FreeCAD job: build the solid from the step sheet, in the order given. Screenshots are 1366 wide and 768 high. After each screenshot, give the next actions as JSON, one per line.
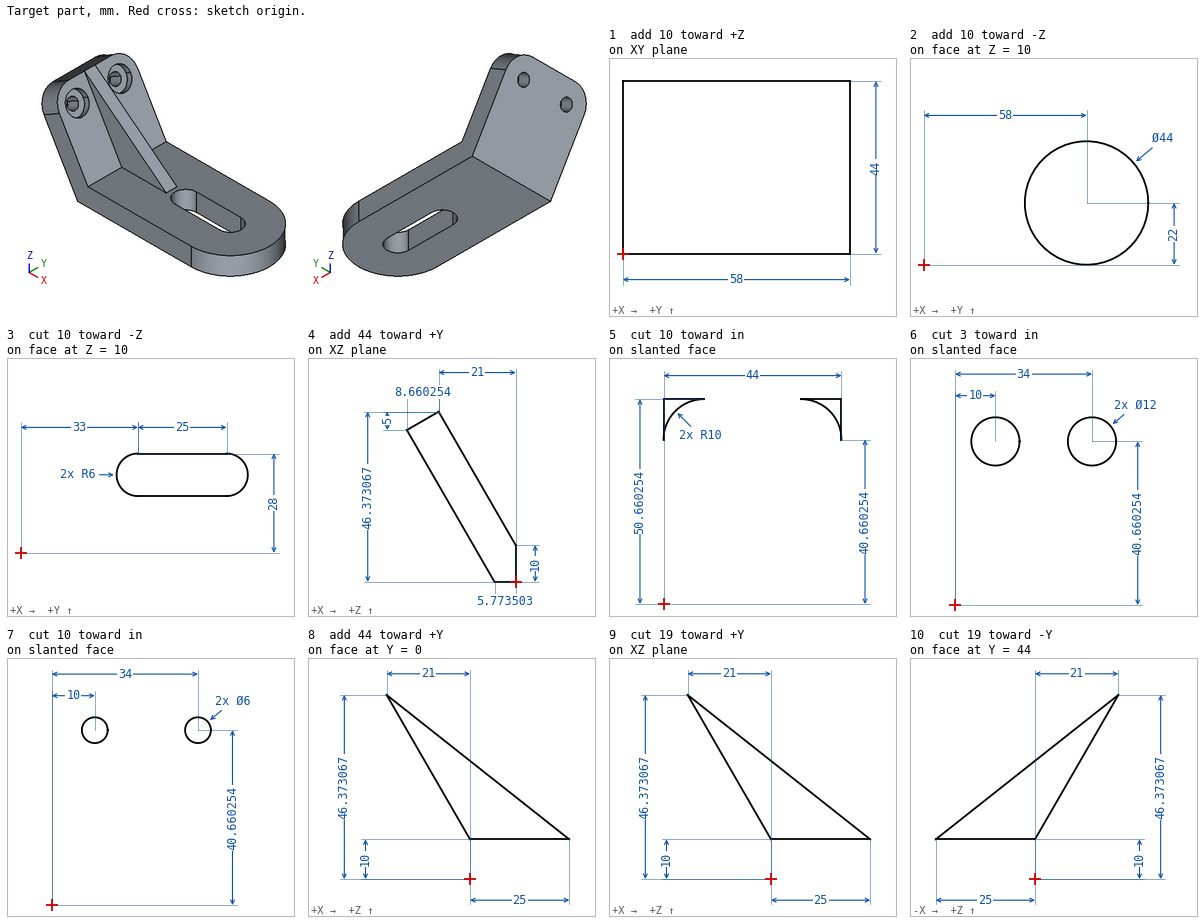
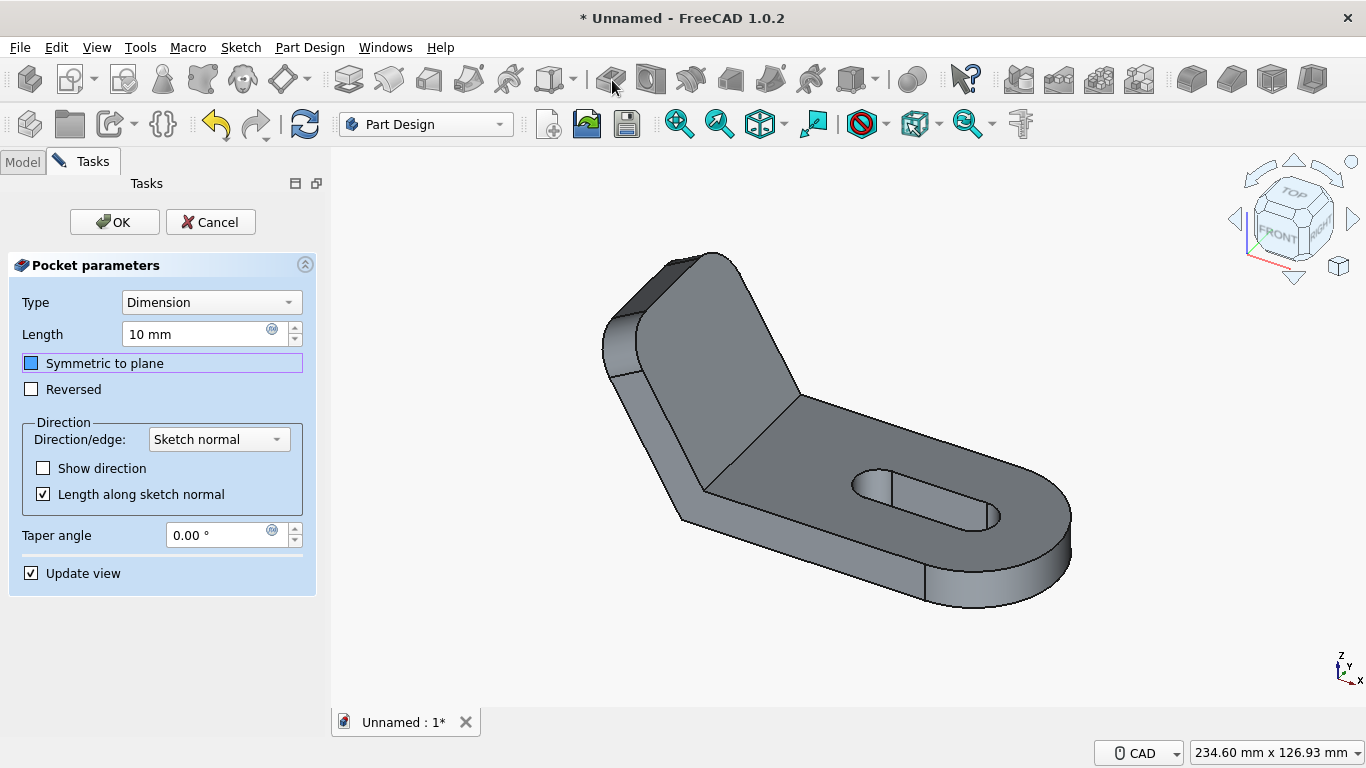
{"action": "left_click", "coordinate": [115, 222]}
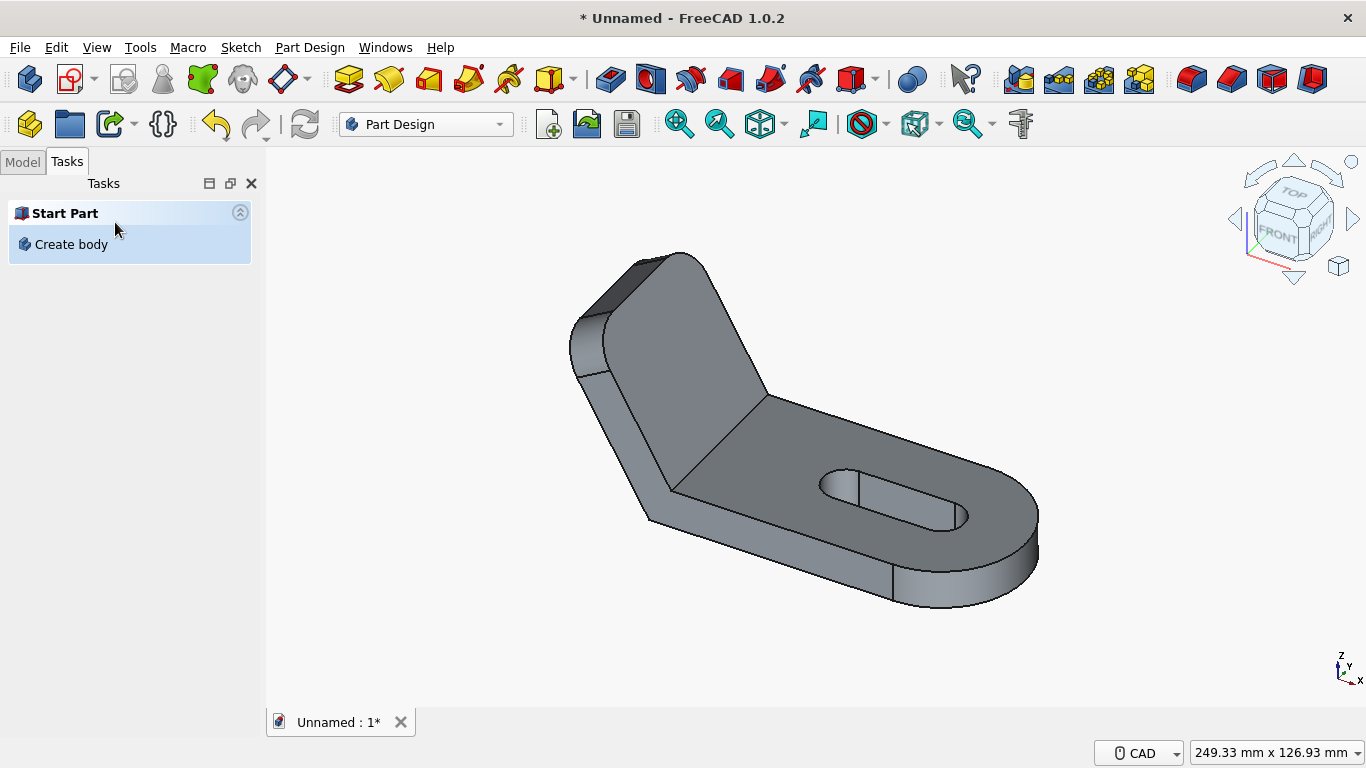
{"action": "left_click", "coordinate": [680, 363]}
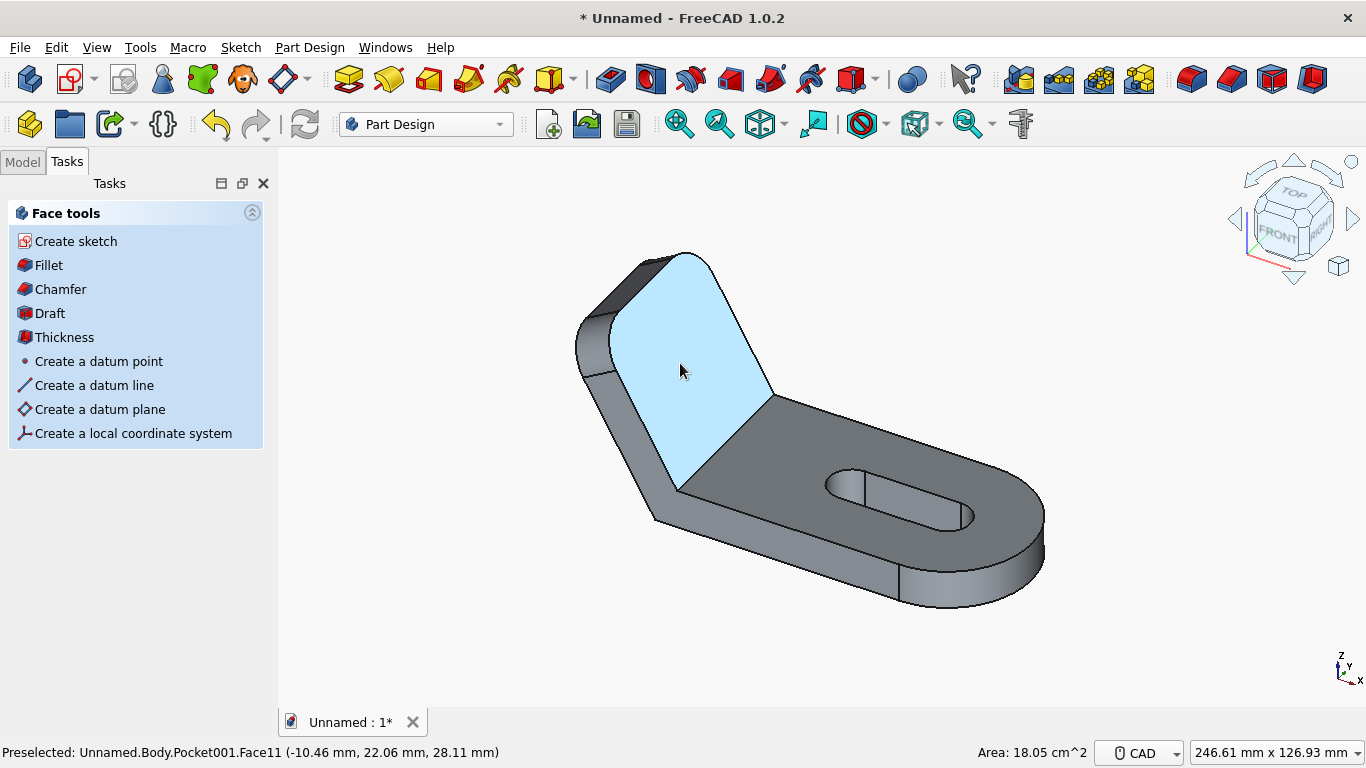
{"action": "left_click", "coordinate": [70, 80]}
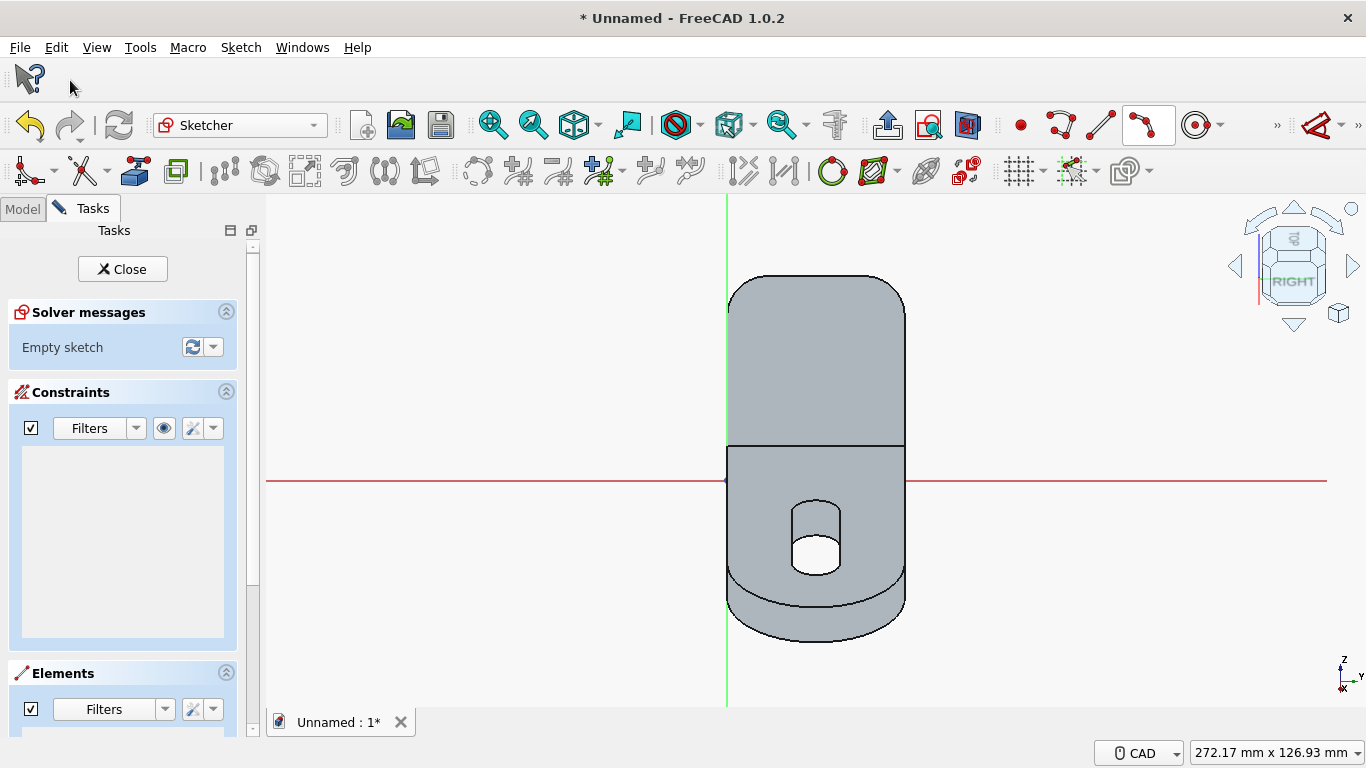
{"action": "scroll", "coordinate": [881, 309], "scroll_direction": "up", "scroll_amount": 3}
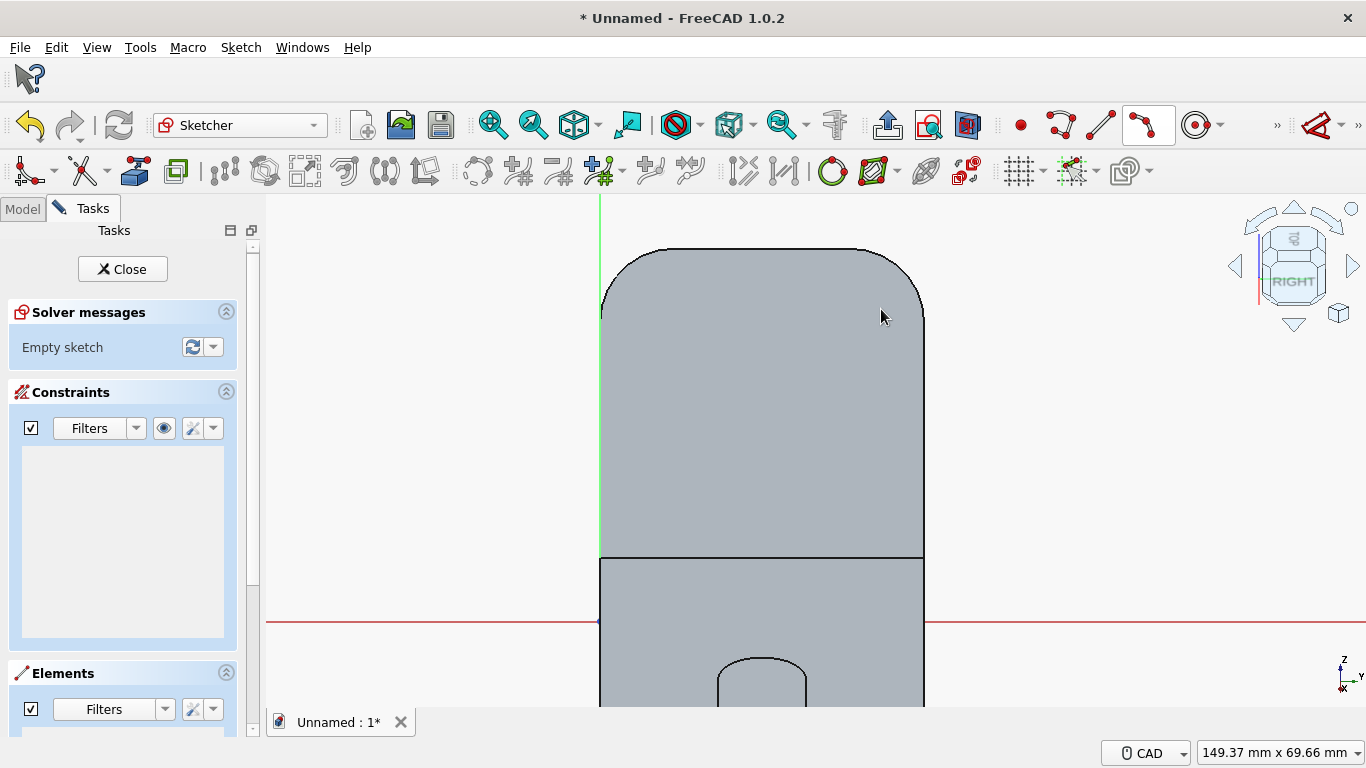
{"action": "left_click", "coordinate": [1196, 126]}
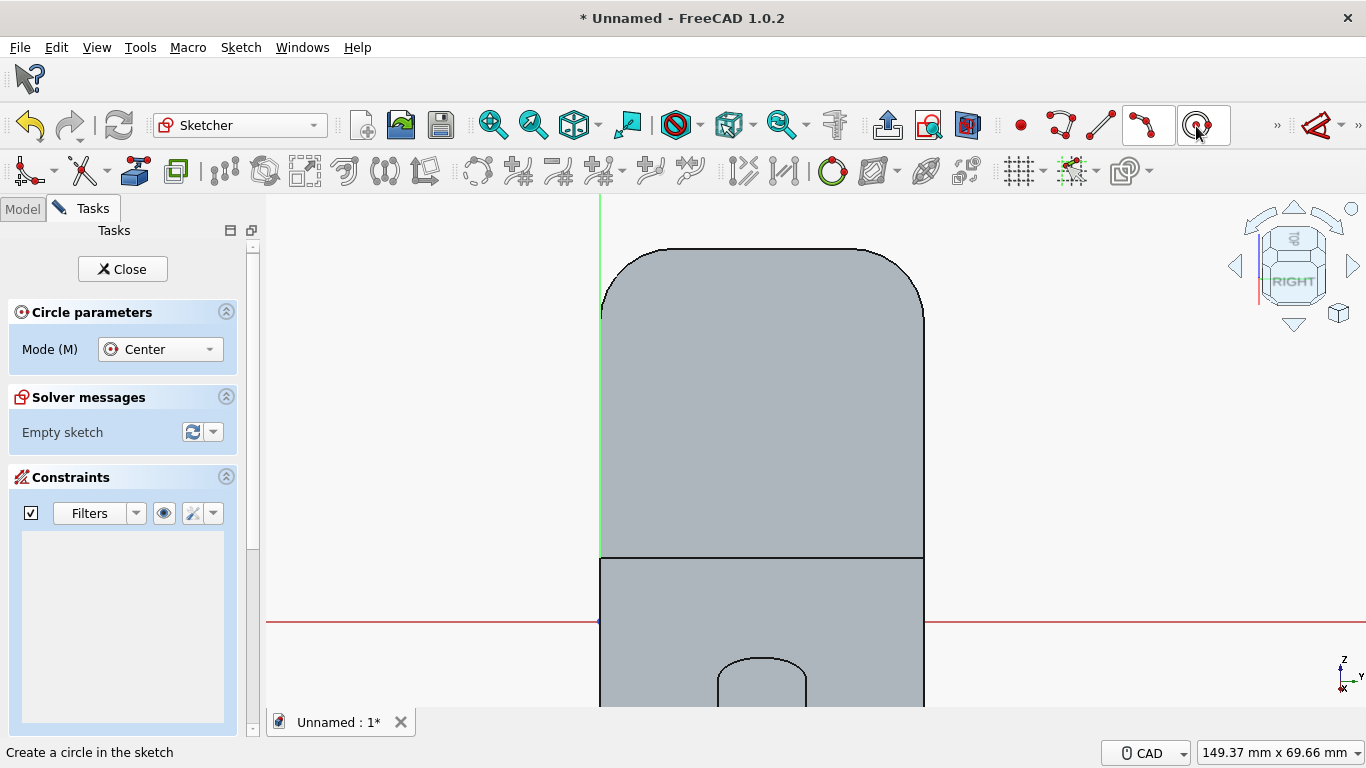
{"action": "left_click", "coordinate": [850, 322]}
{"action": "mouse_move", "coordinate": [882, 291]}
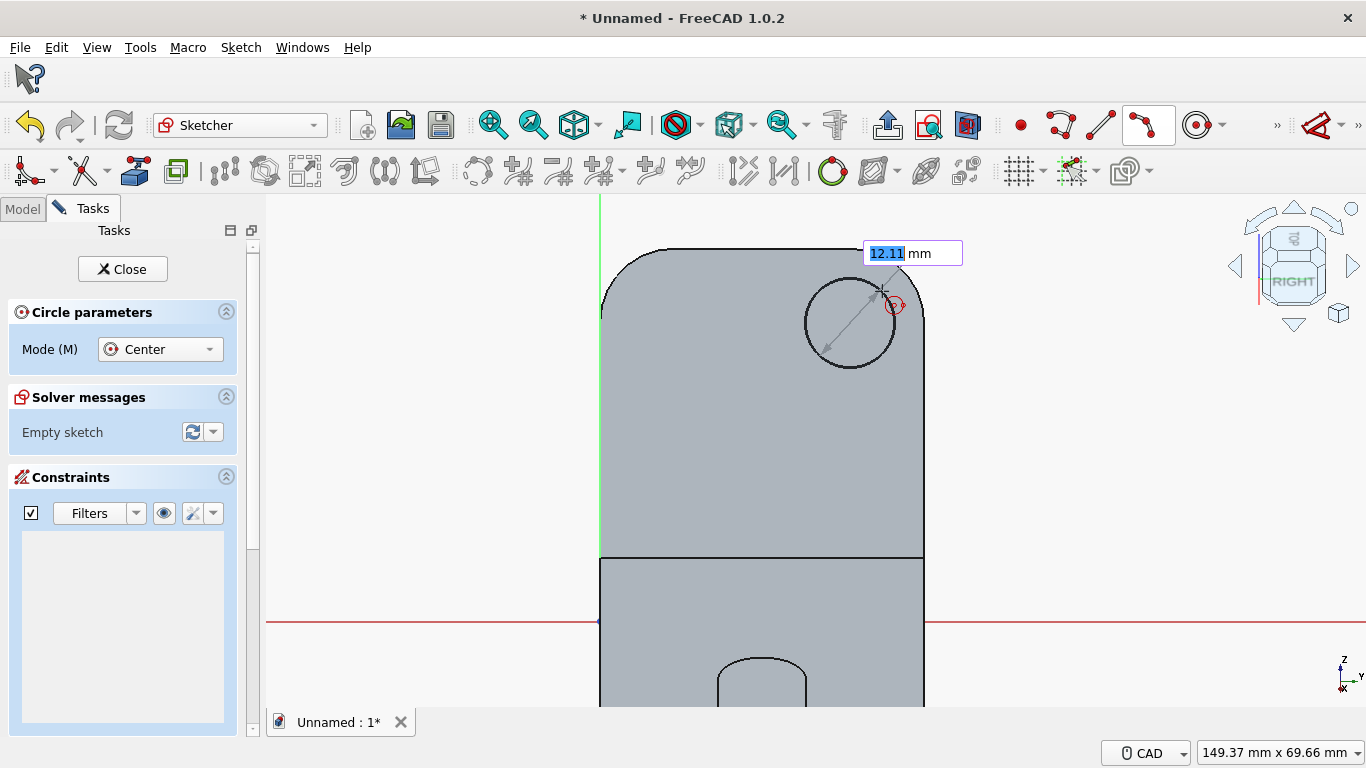
{"action": "type", "text": "12"}
{"action": "key", "text": "Return"}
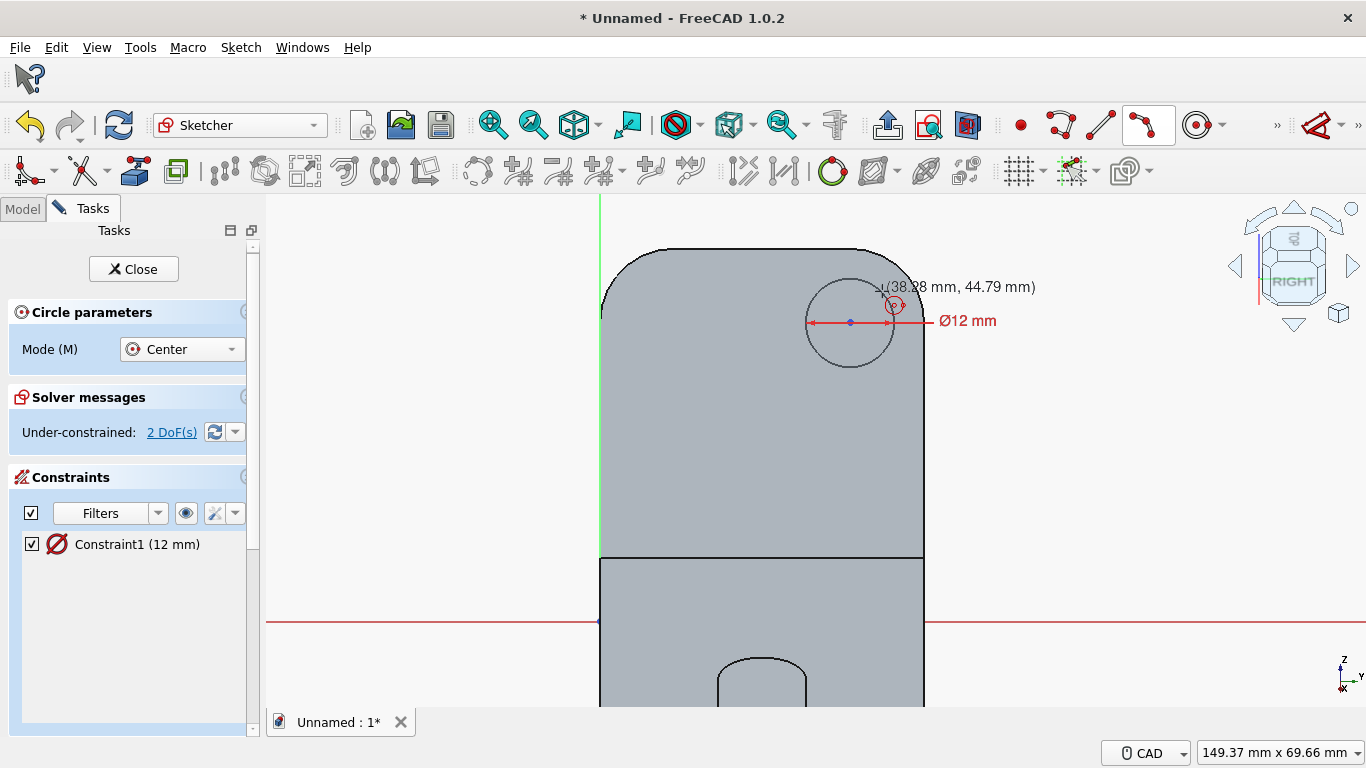
{"action": "left_click", "coordinate": [674, 322]}
{"action": "mouse_move", "coordinate": [705, 291]}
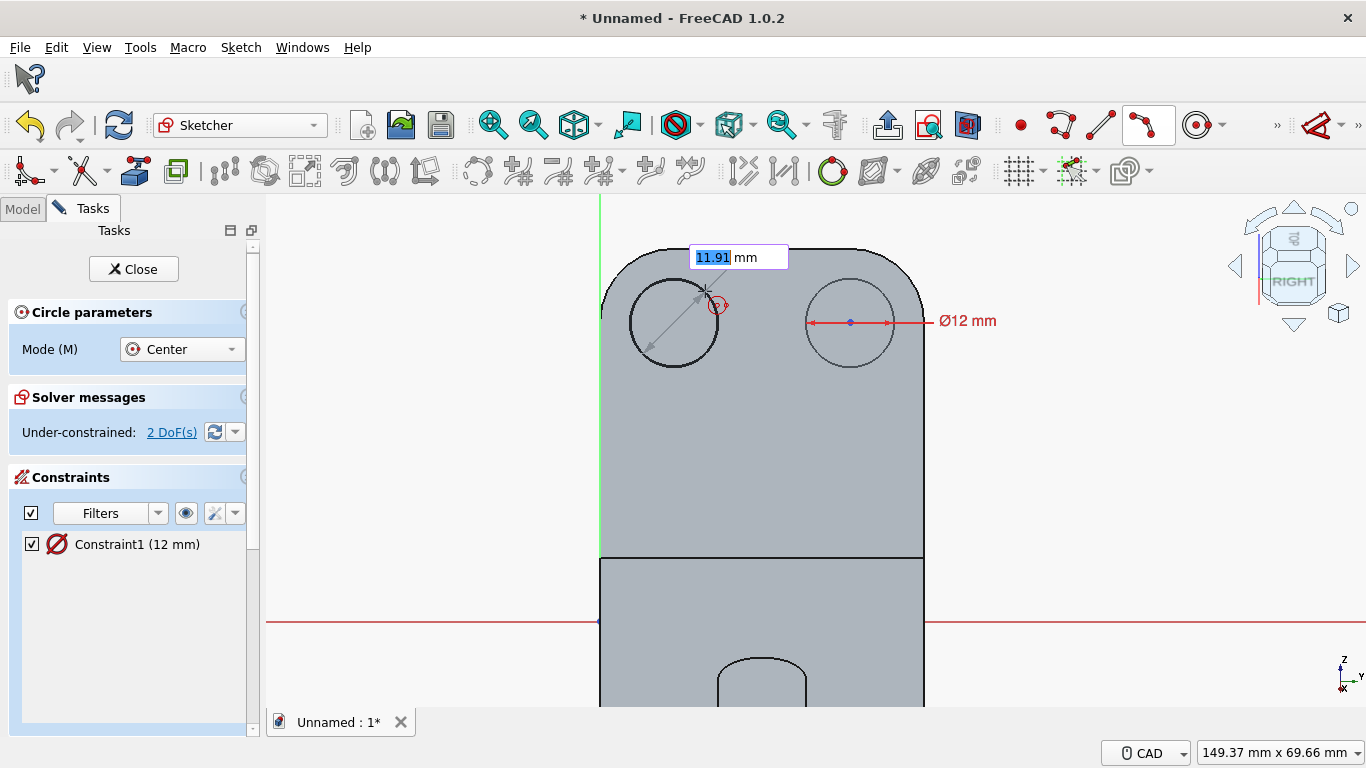
{"action": "type", "text": "12"}
{"action": "key", "text": "Return"}
{"action": "key", "text": "Escape"}